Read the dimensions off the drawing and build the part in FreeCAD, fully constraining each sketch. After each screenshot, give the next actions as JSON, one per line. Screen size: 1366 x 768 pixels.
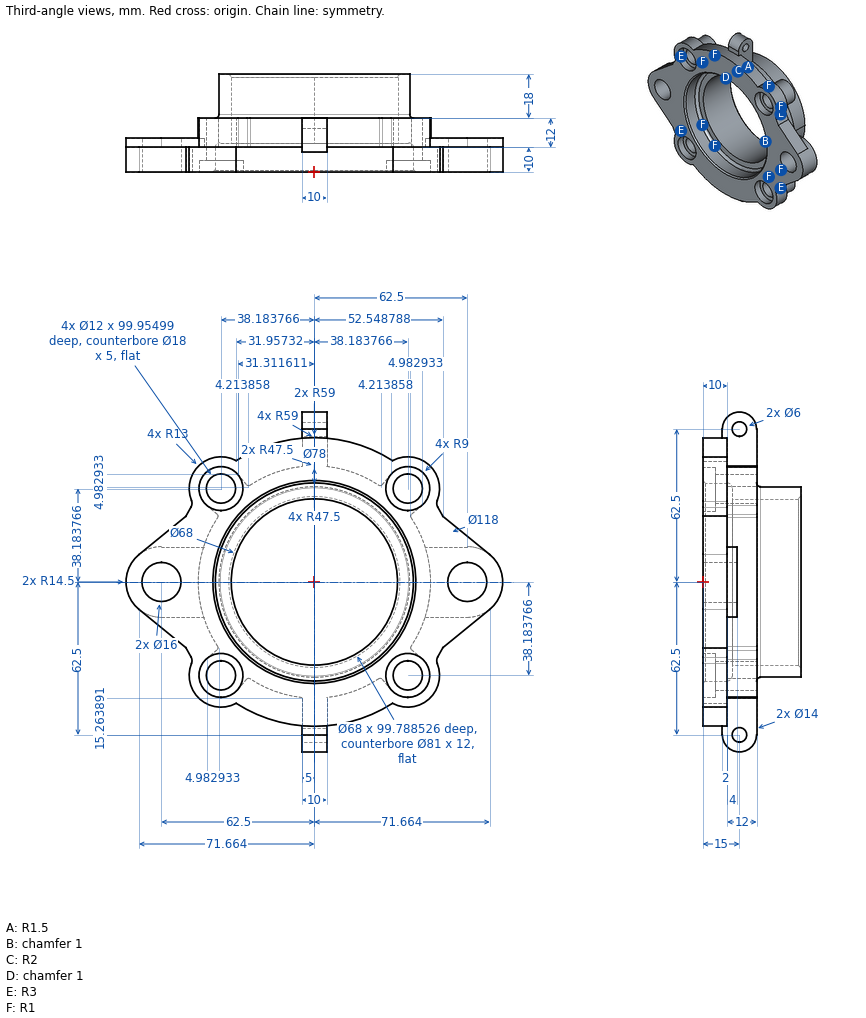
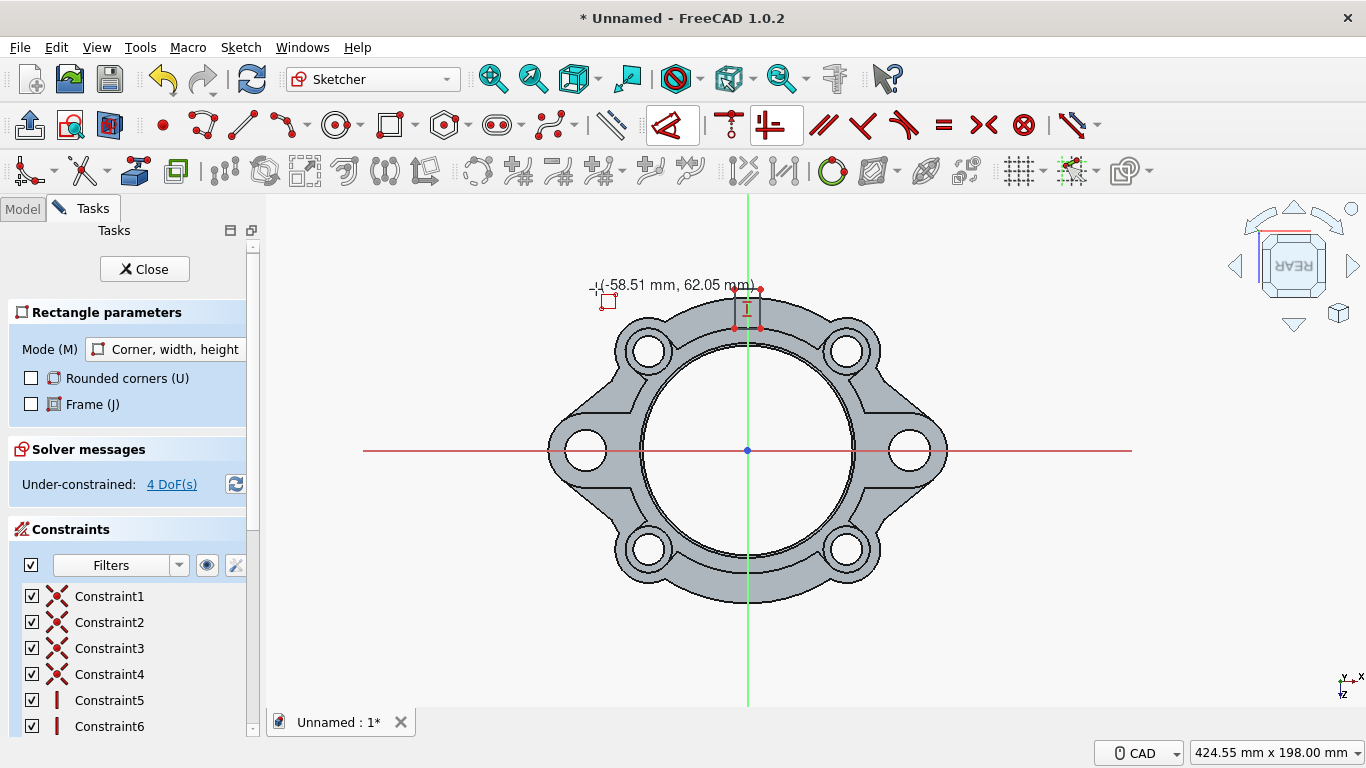
{"action": "scroll", "coordinate": [735, 573], "scroll_direction": "up", "scroll_amount": 2}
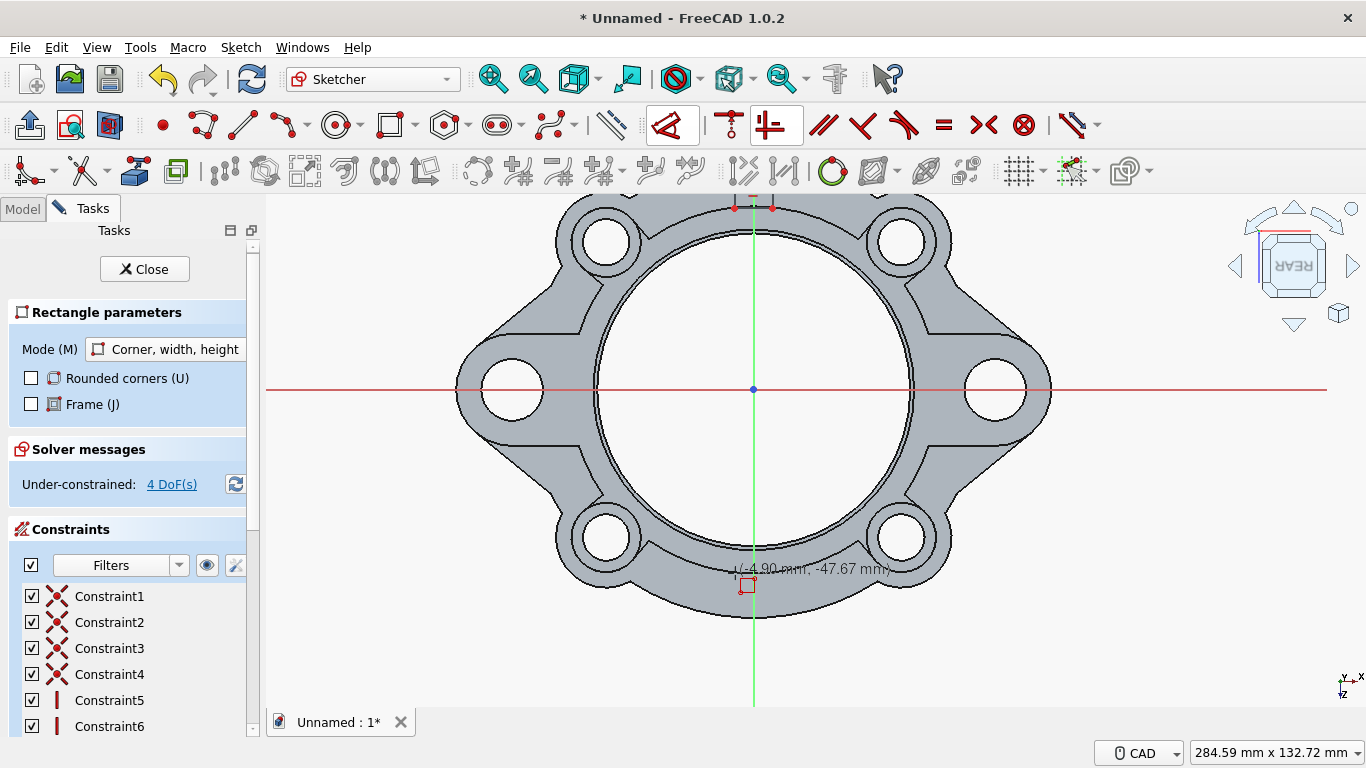
{"action": "left_click", "coordinate": [734, 572]}
{"action": "left_click", "coordinate": [773, 631]}
{"action": "key", "text": "Escape"}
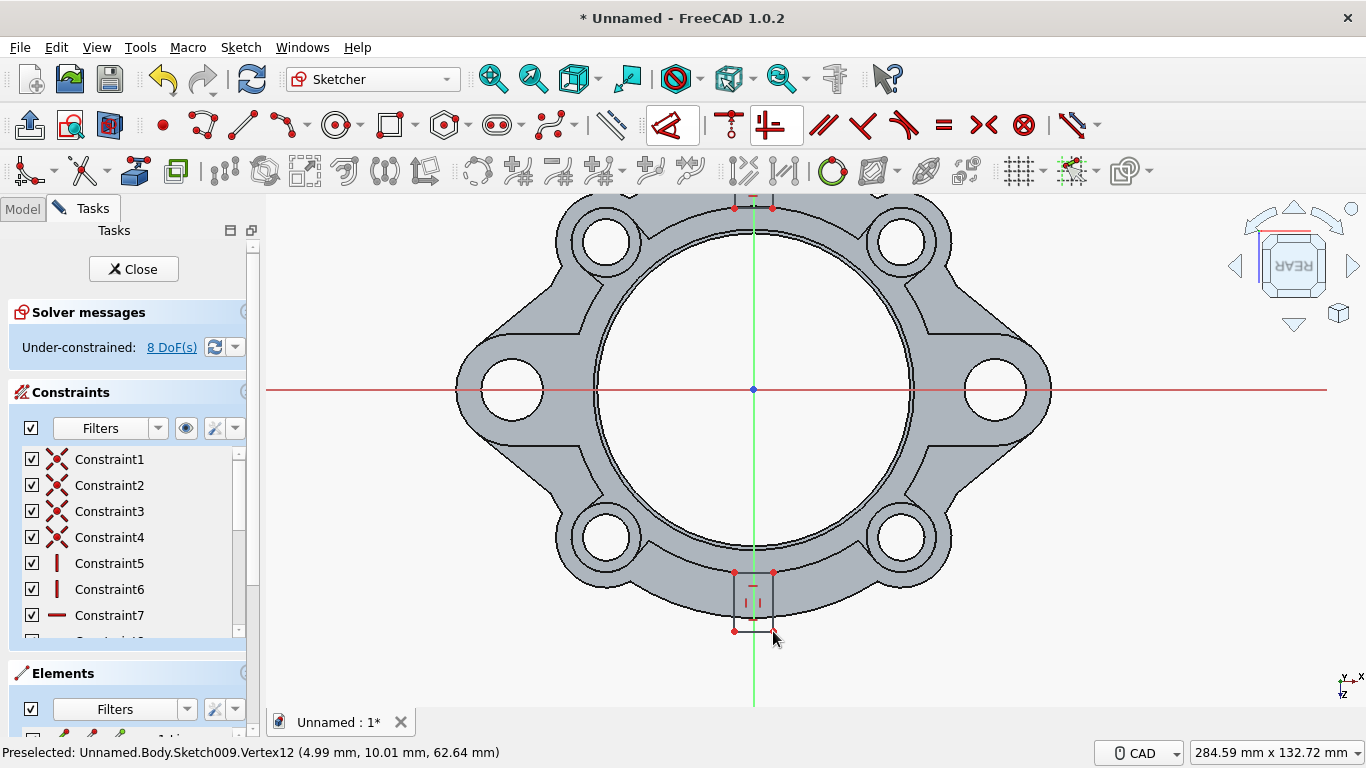
{"action": "scroll", "coordinate": [735, 574], "scroll_direction": "down", "scroll_amount": 2}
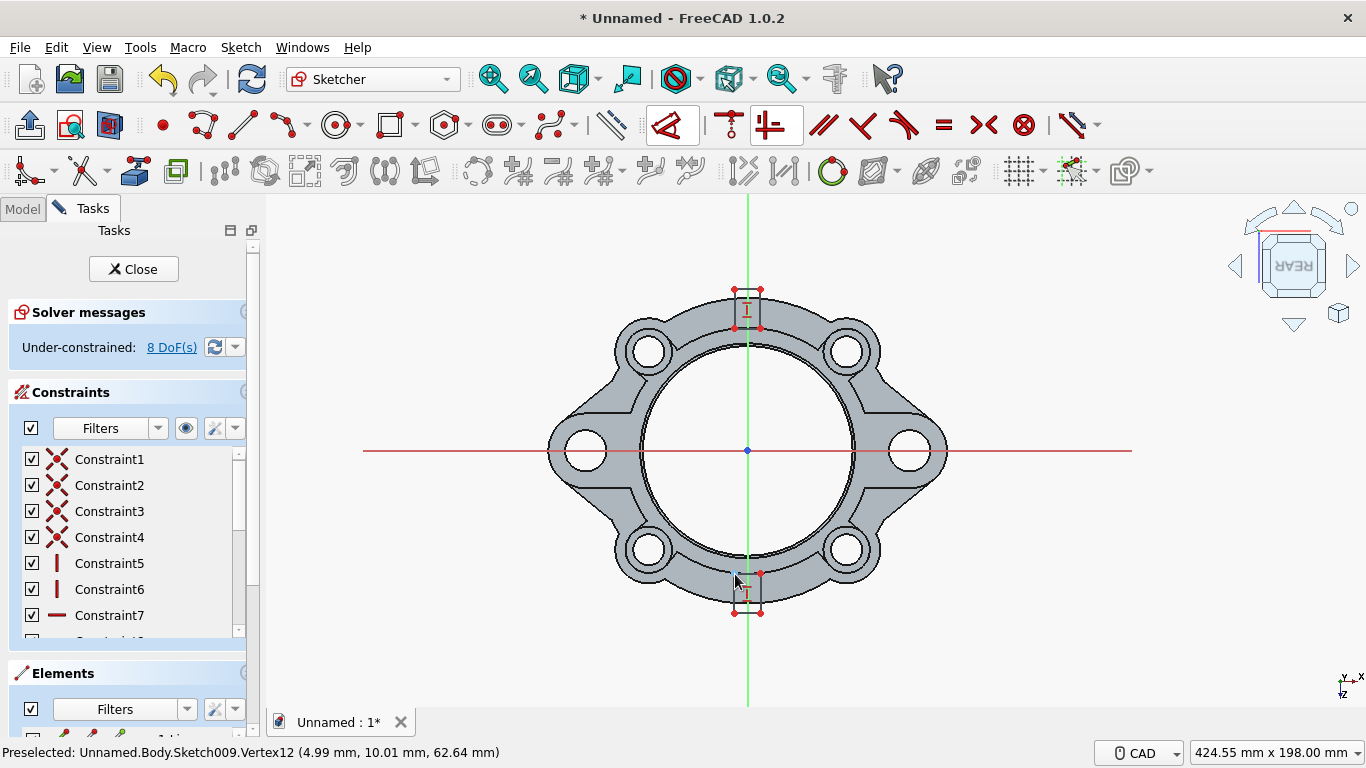
{"action": "left_click", "coordinate": [735, 329]}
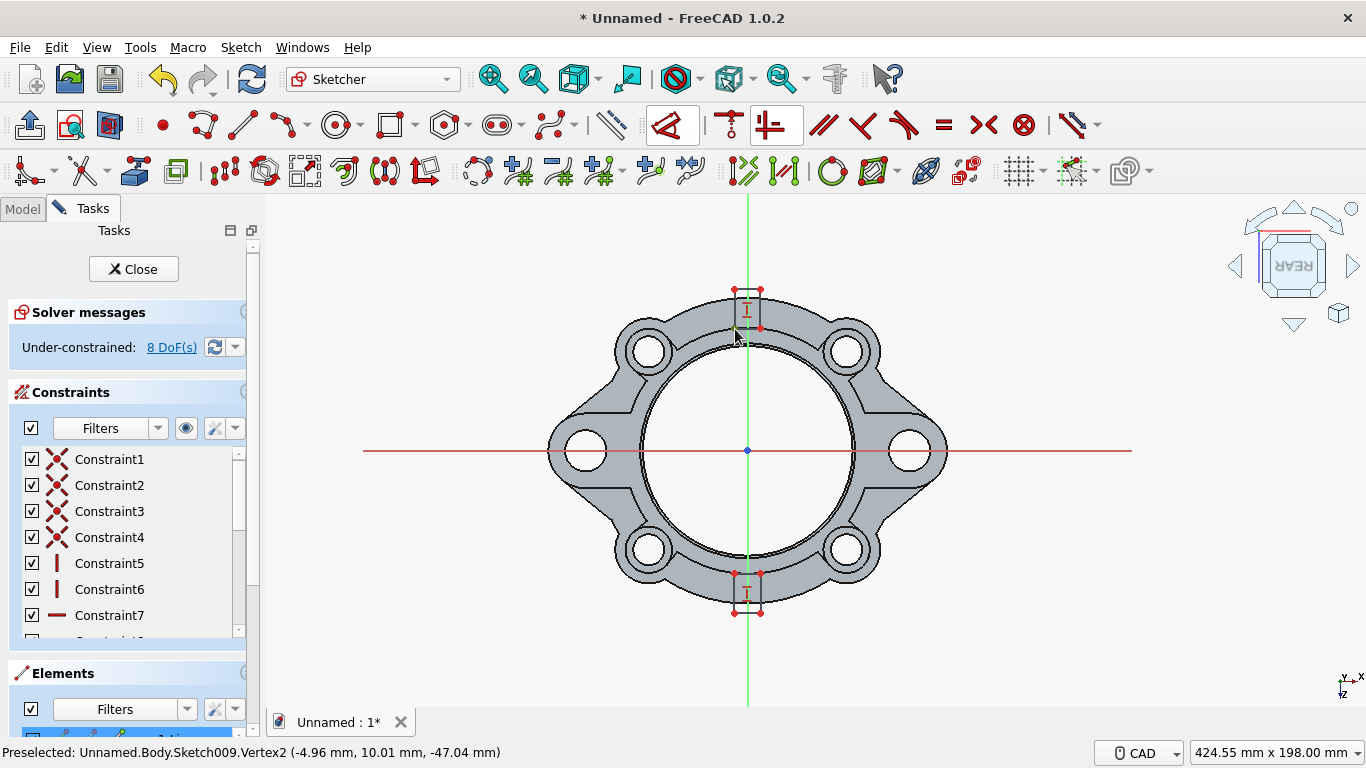
{"action": "left_click", "coordinate": [734, 574]}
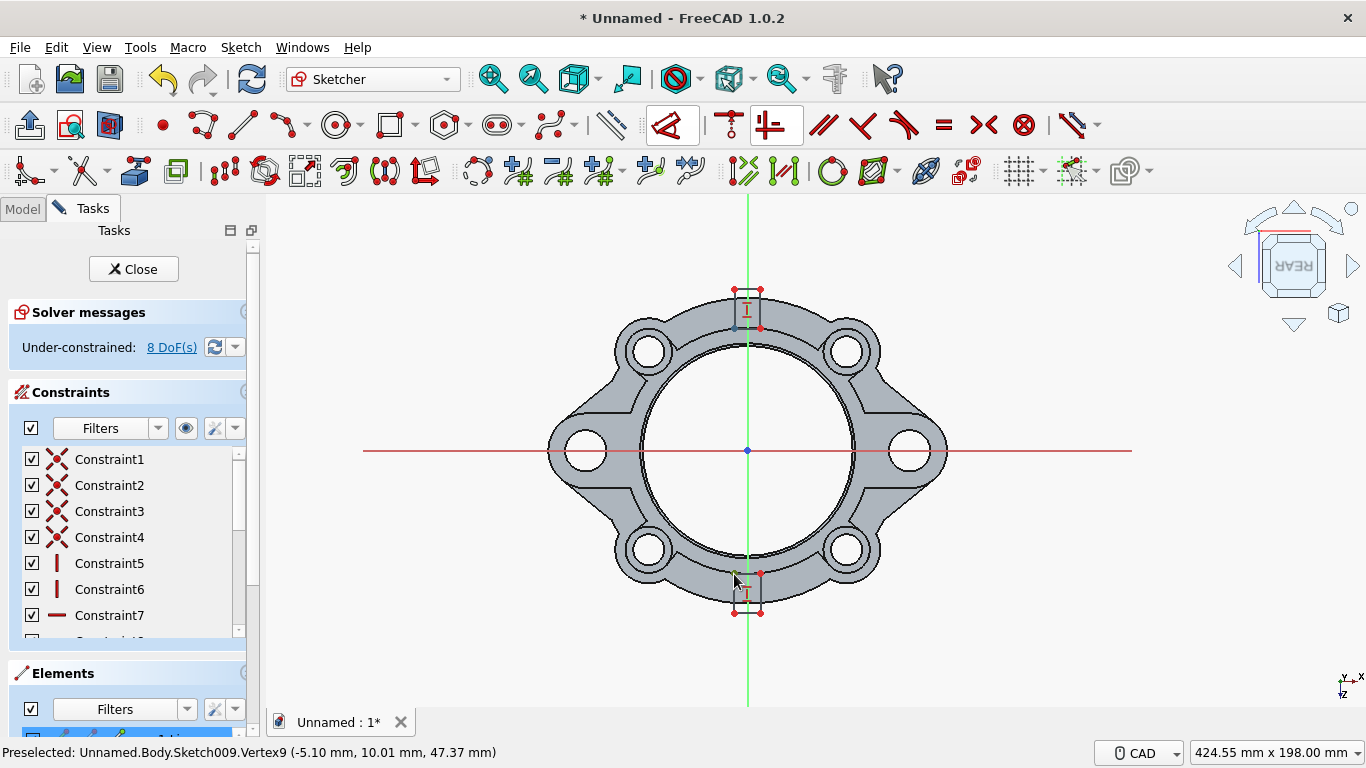
{"action": "left_click", "coordinate": [359, 451]}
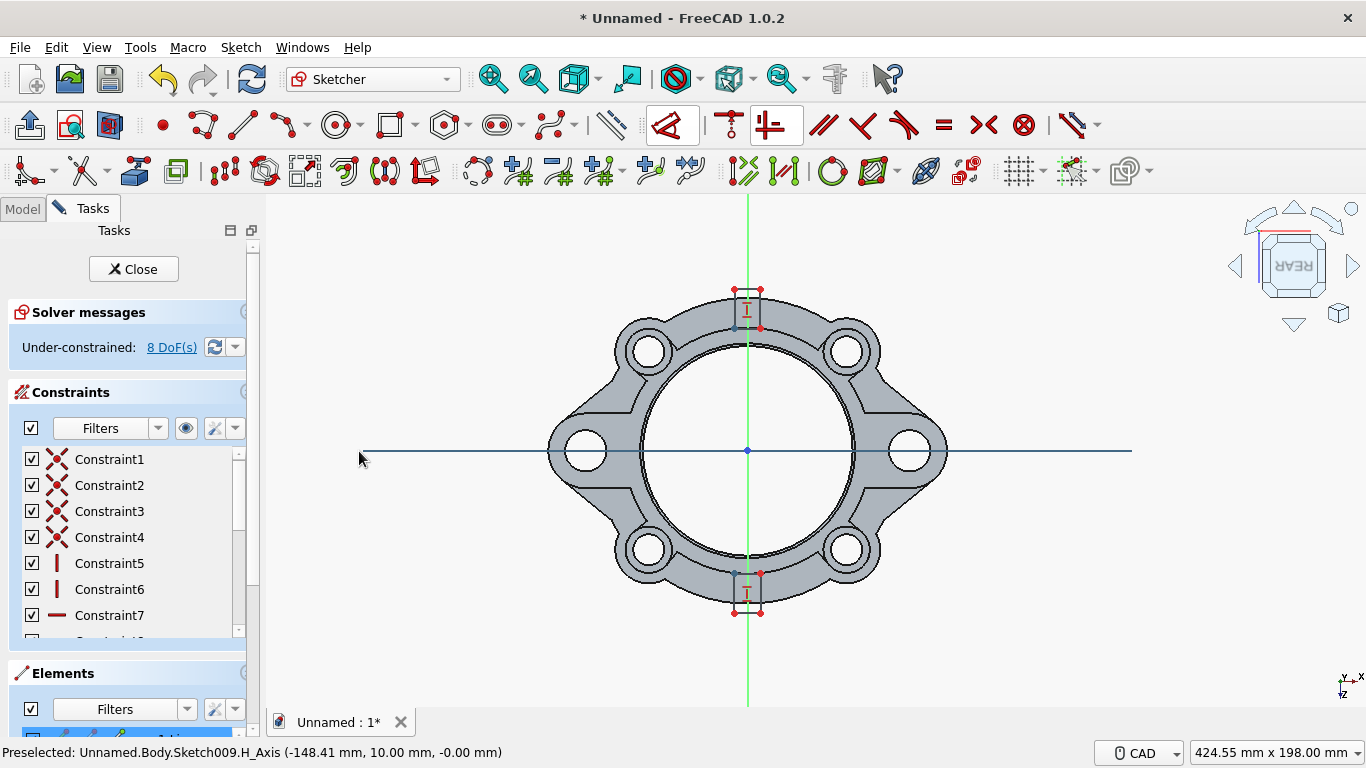
{"action": "left_click", "coordinate": [984, 126]}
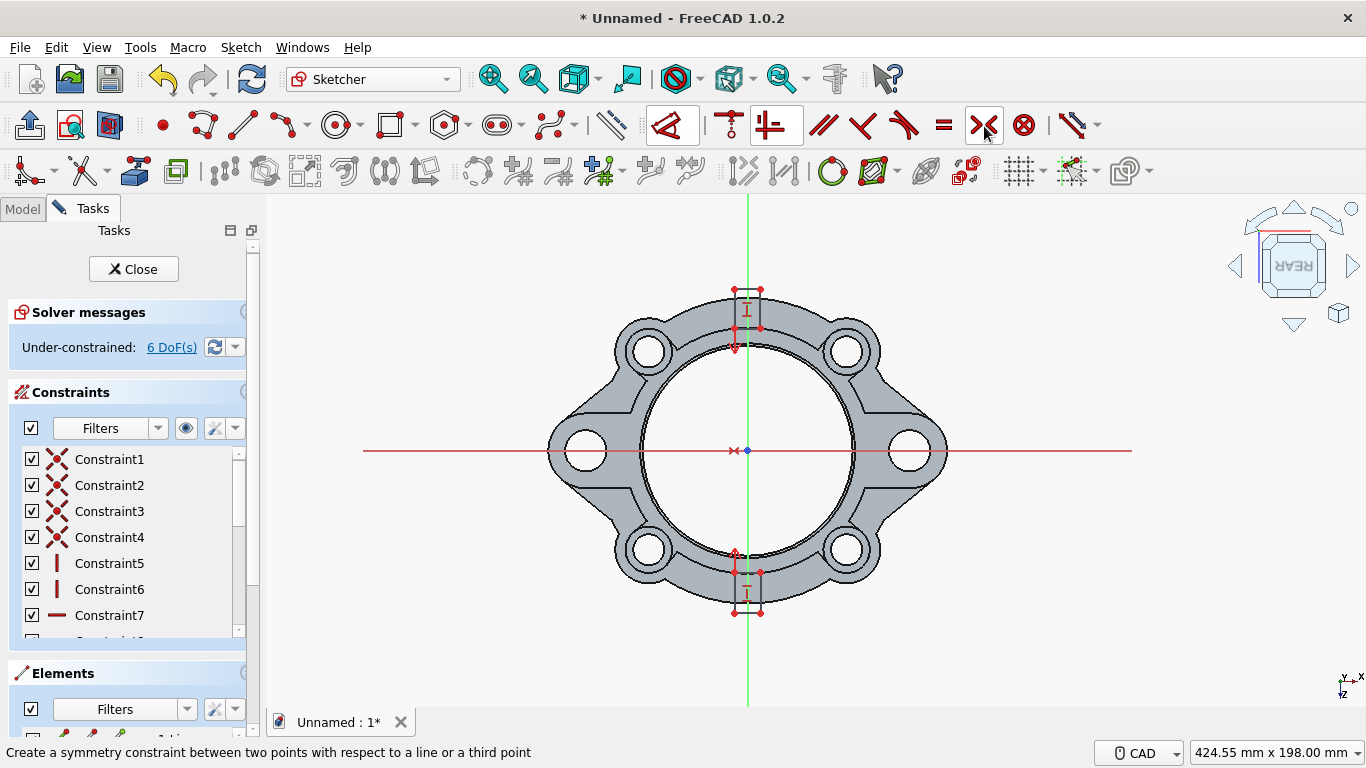
{"action": "left_click", "coordinate": [760, 289]}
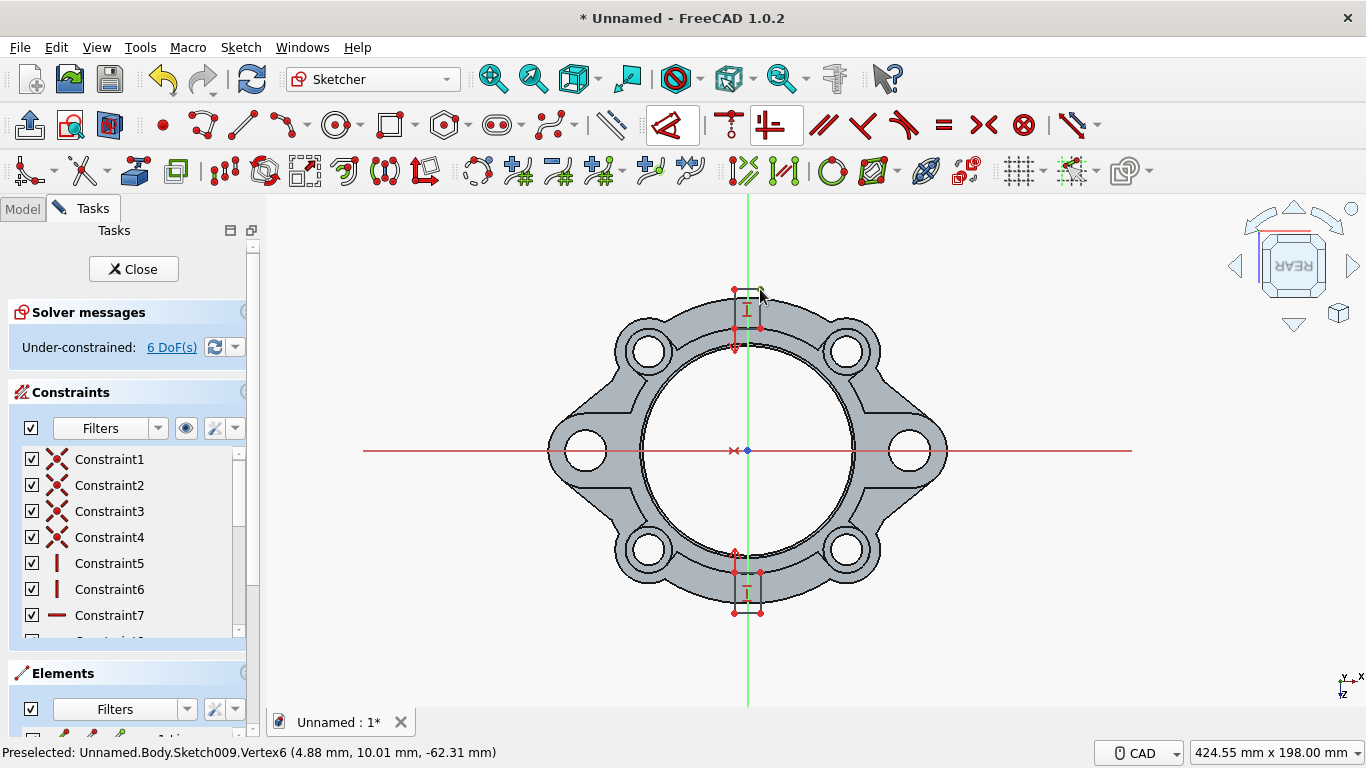
{"action": "left_click", "coordinate": [761, 613]}